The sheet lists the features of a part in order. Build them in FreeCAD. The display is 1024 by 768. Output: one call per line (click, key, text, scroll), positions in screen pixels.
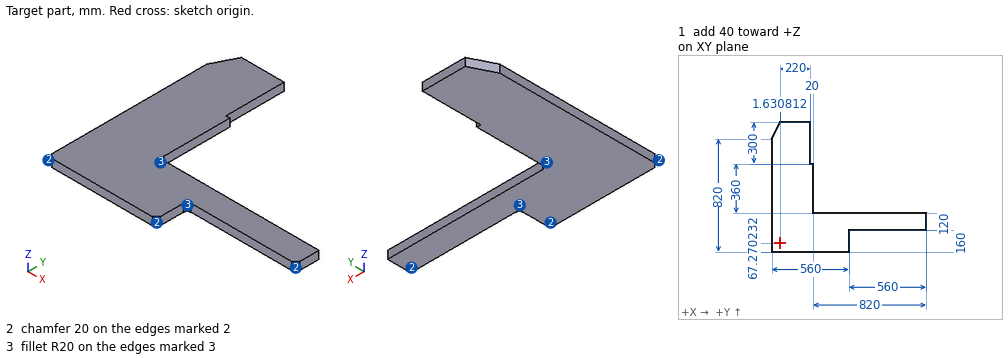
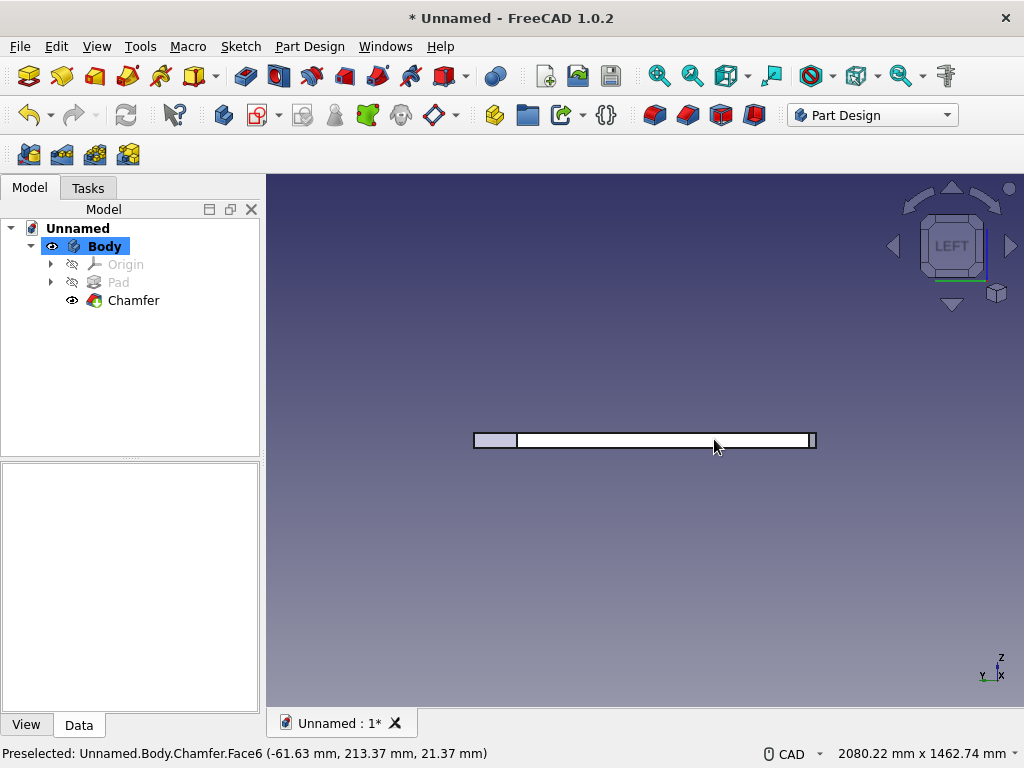
key(v)
key(3)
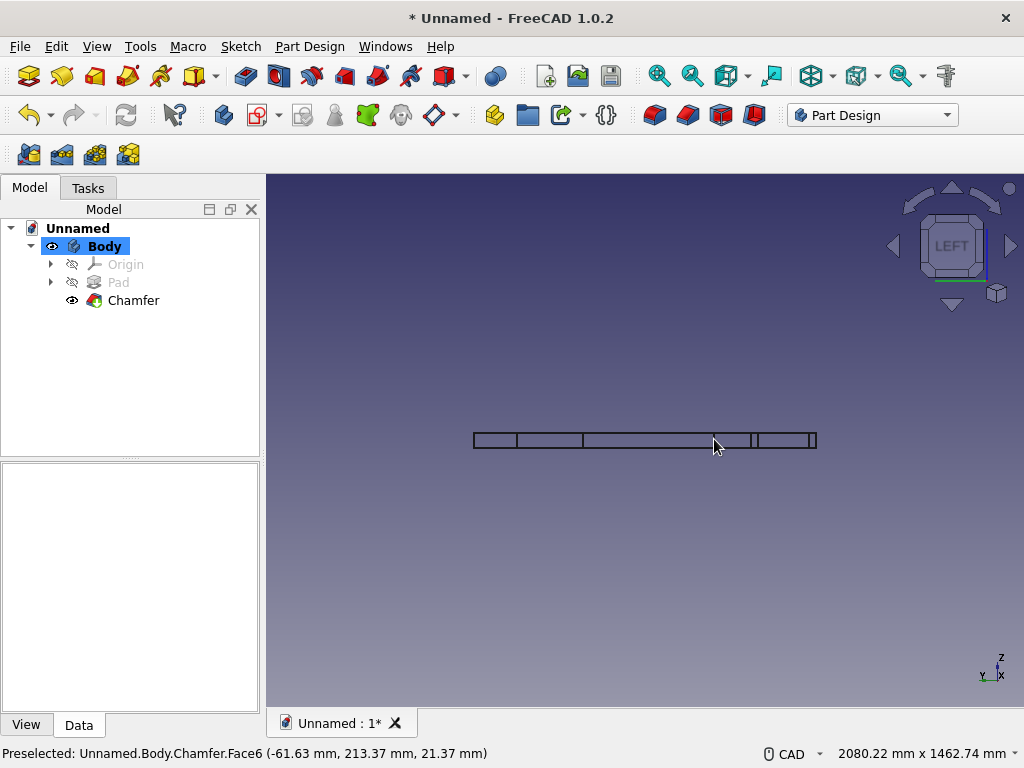
key(0)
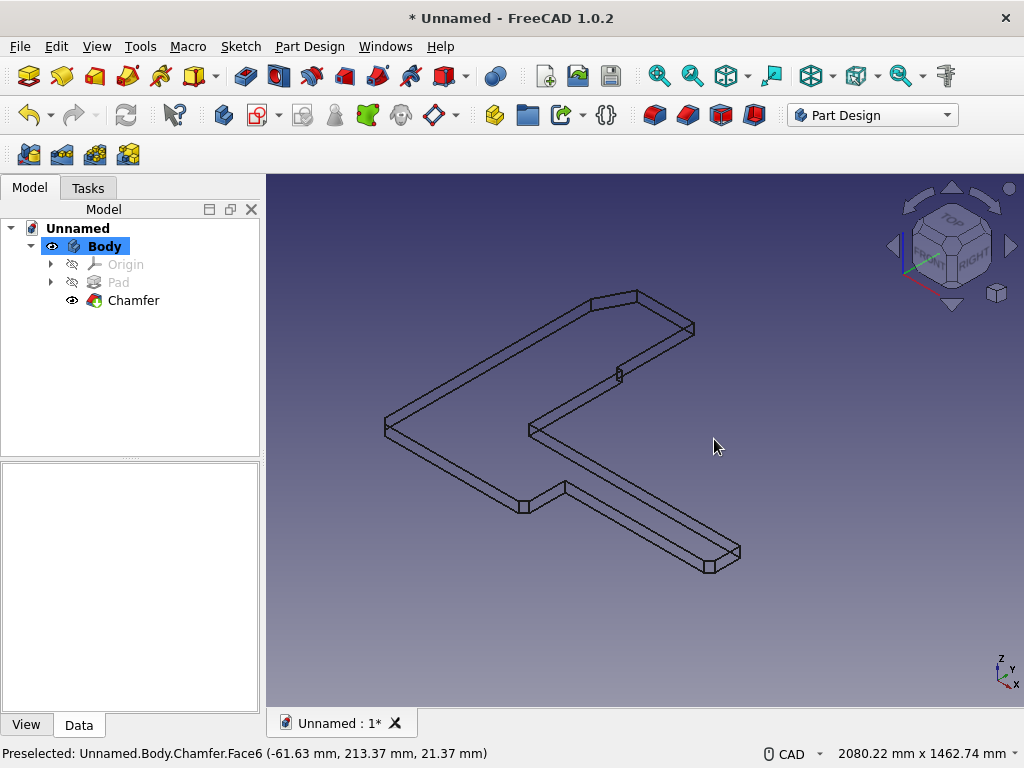
click(529, 431)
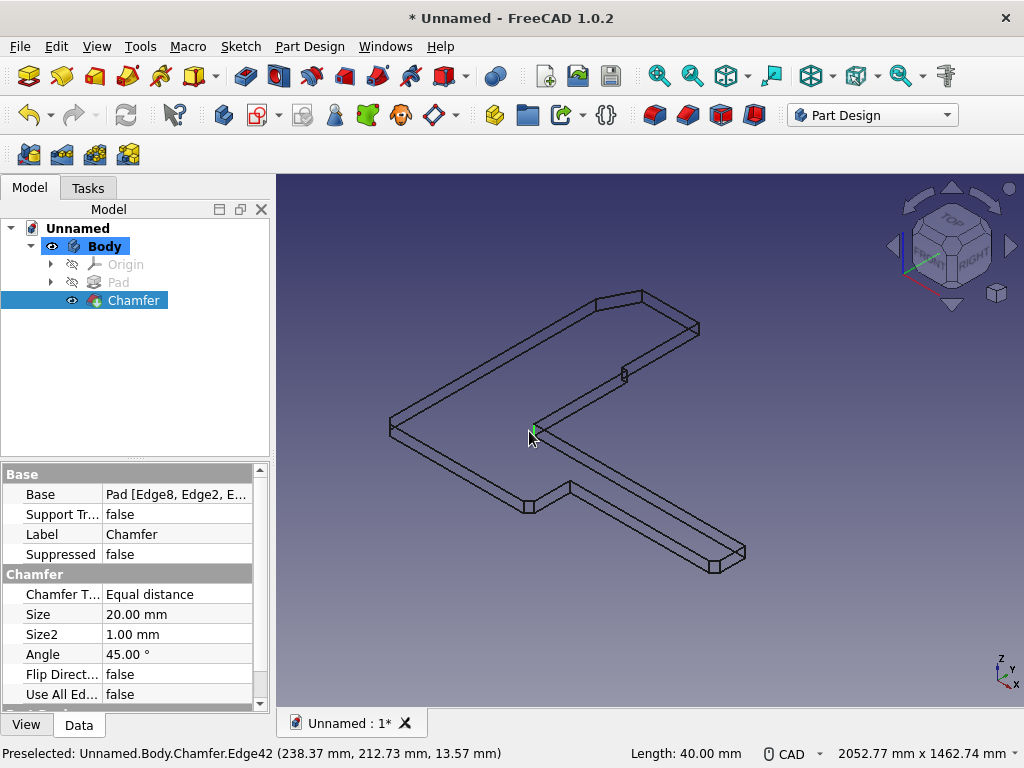
click(570, 488, ctrl)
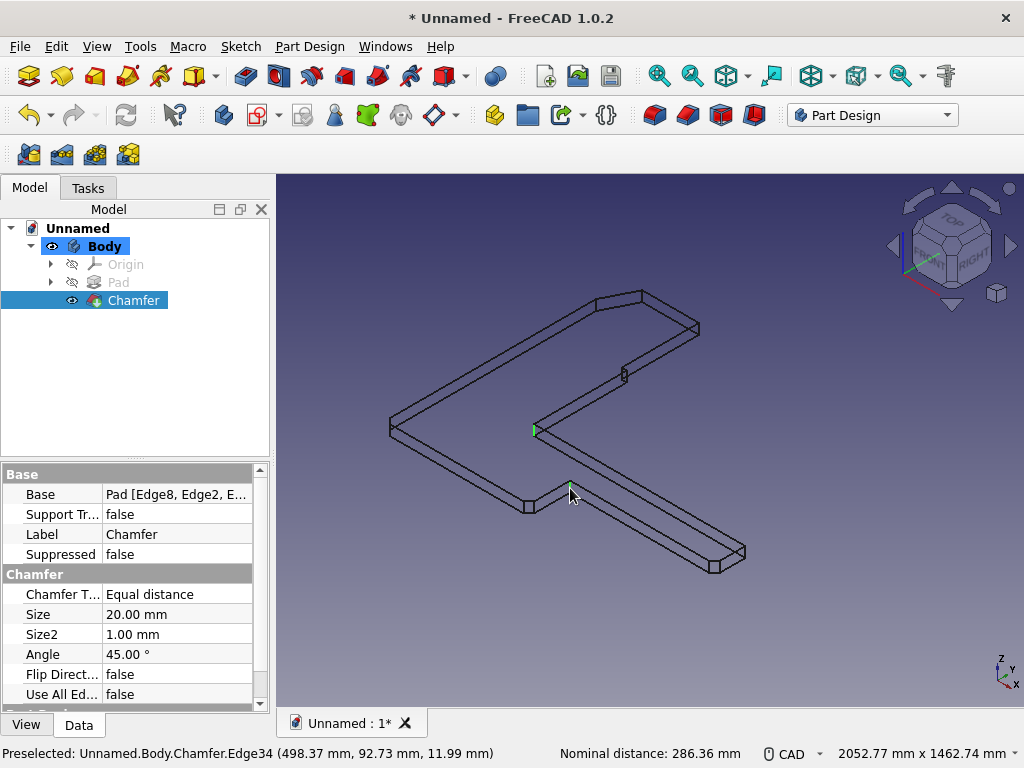
key(v)
key(1)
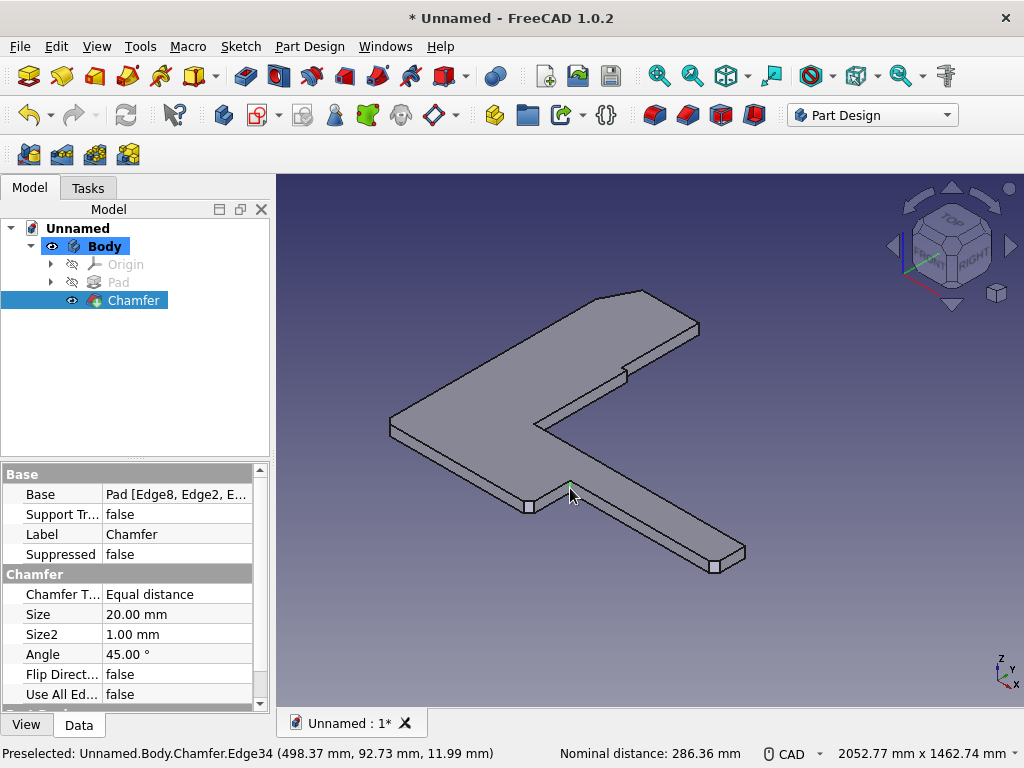
click(655, 116)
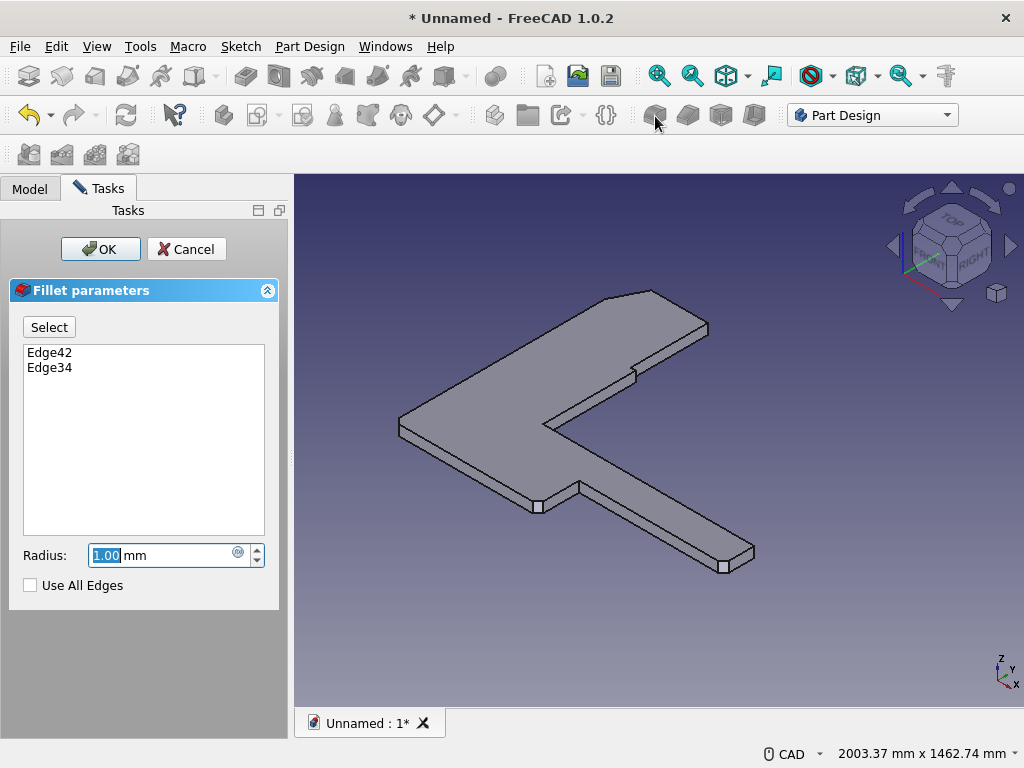
text(20)
key(Tab)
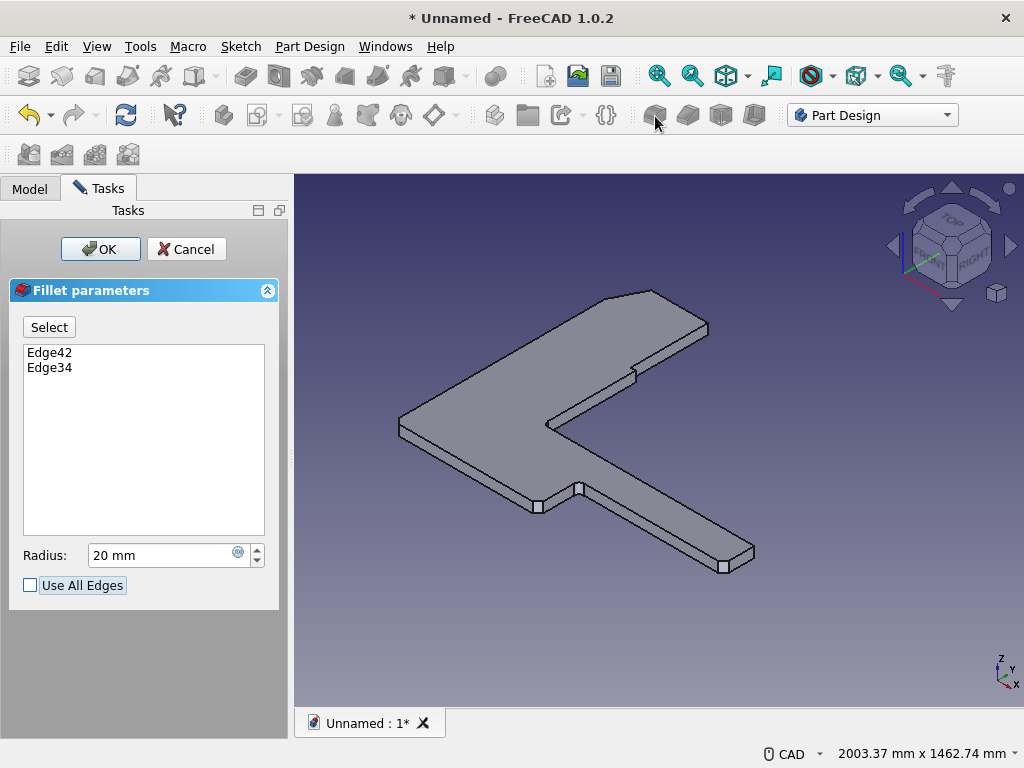
click(101, 249)